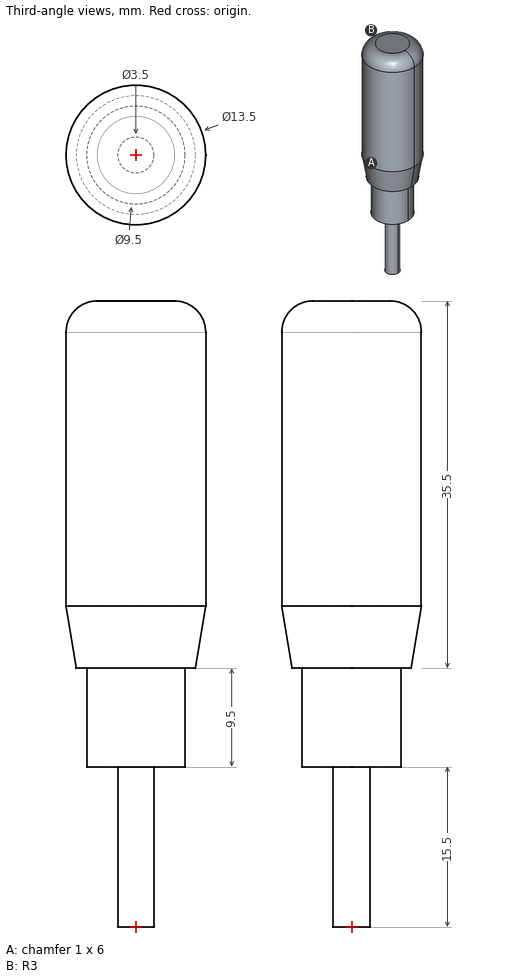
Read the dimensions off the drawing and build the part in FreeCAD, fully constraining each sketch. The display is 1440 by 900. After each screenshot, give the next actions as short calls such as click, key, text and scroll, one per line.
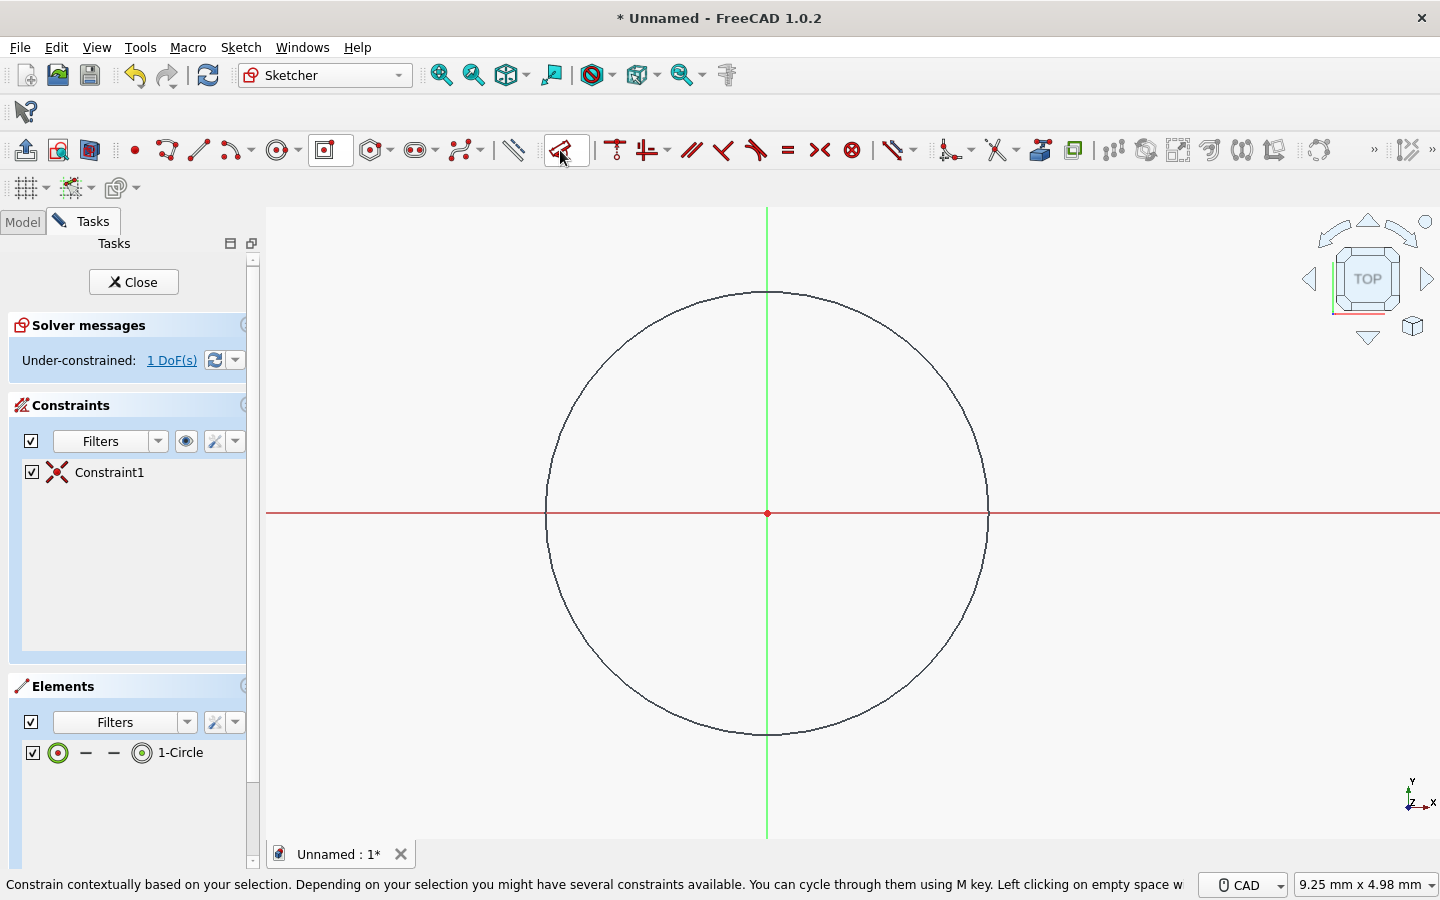
click(923, 356)
click(946, 333)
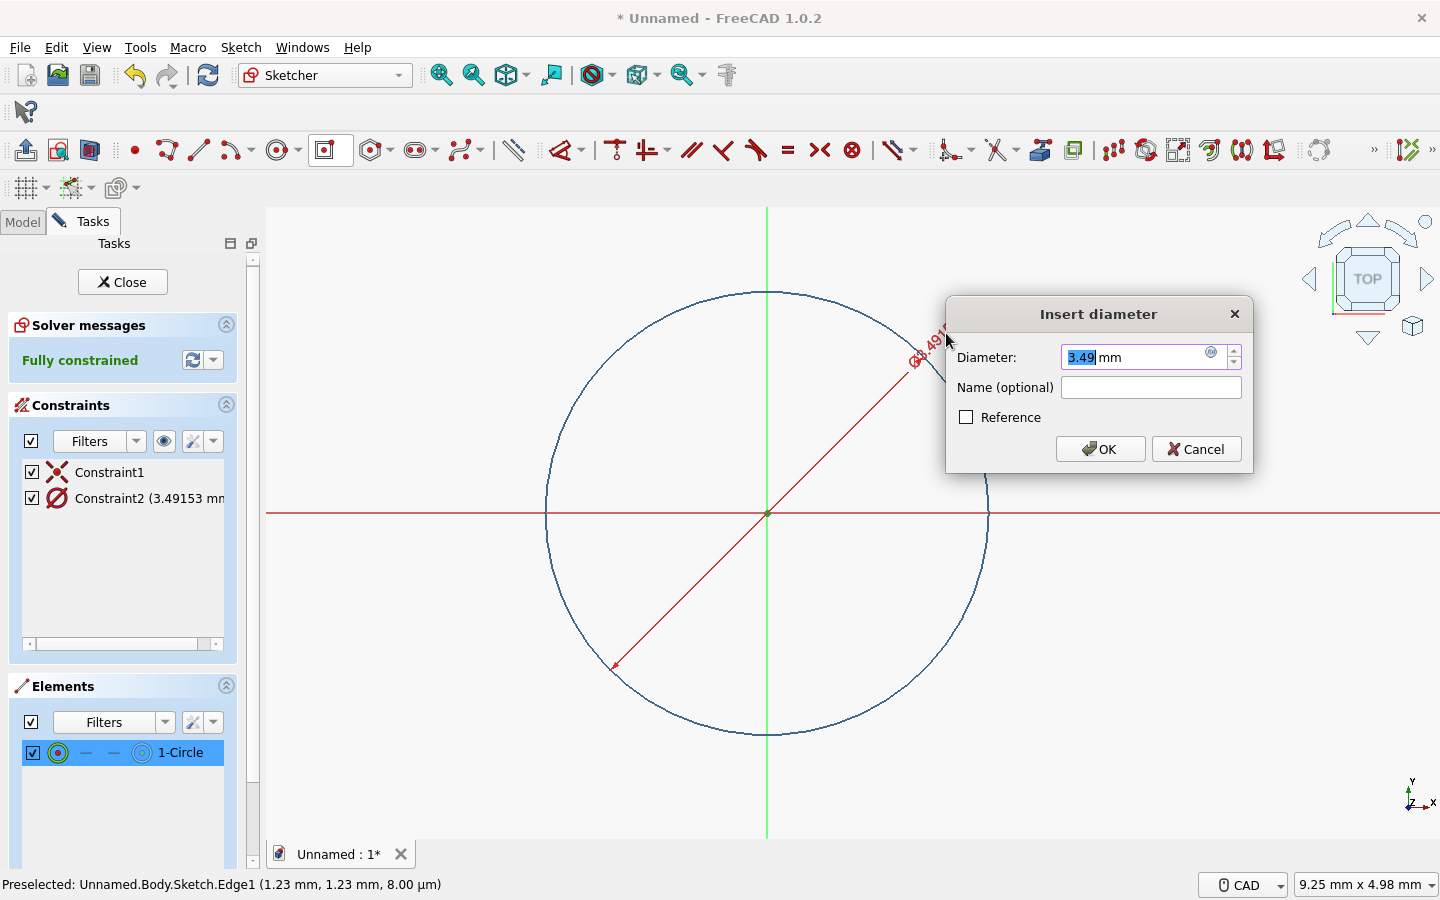
text(3.5)
key(Return)
key(Escape)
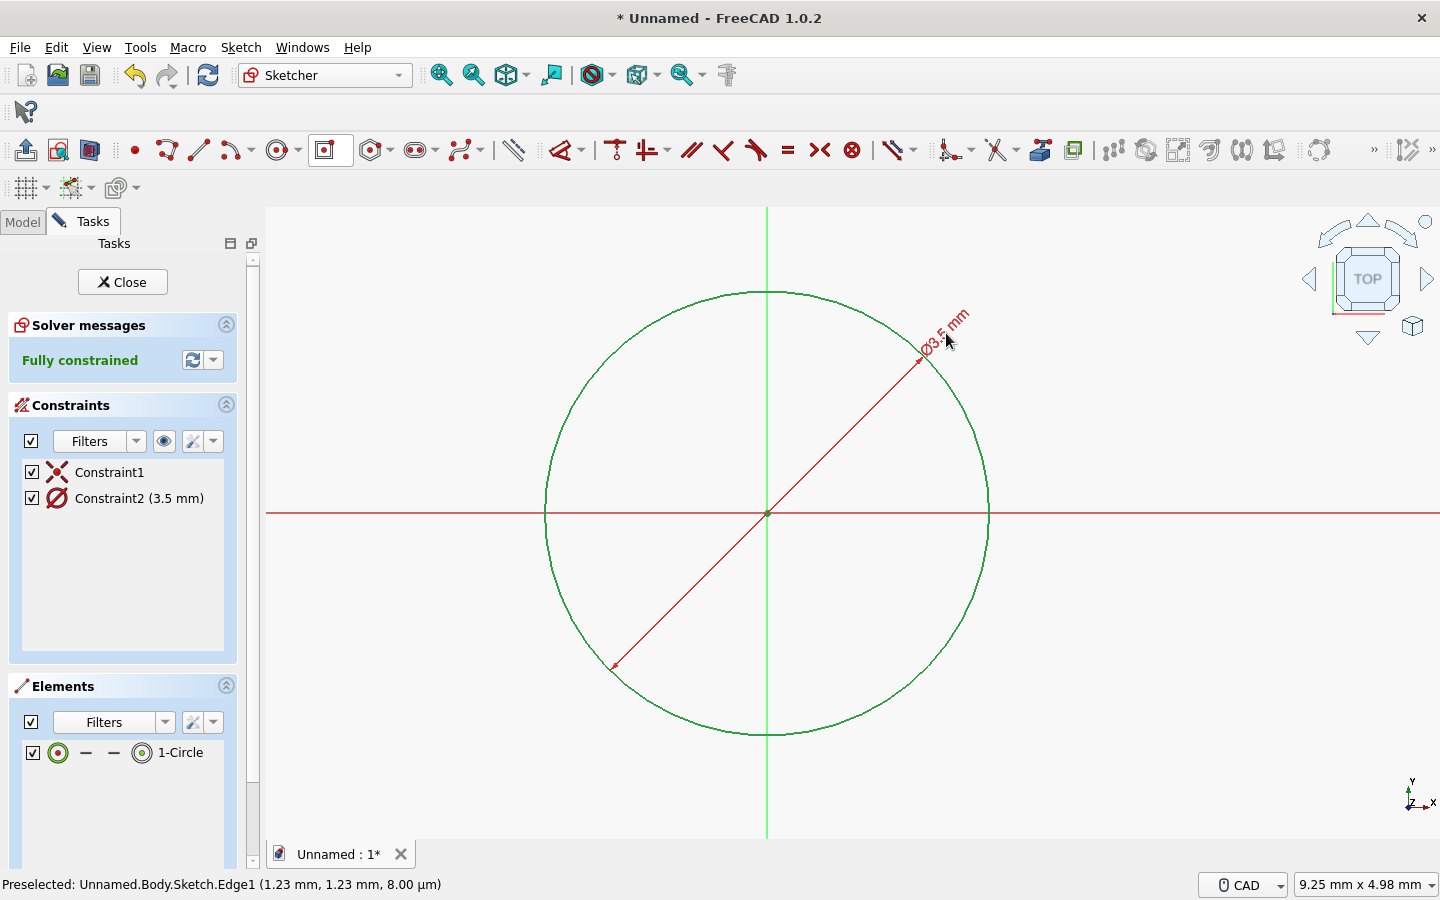
click(123, 282)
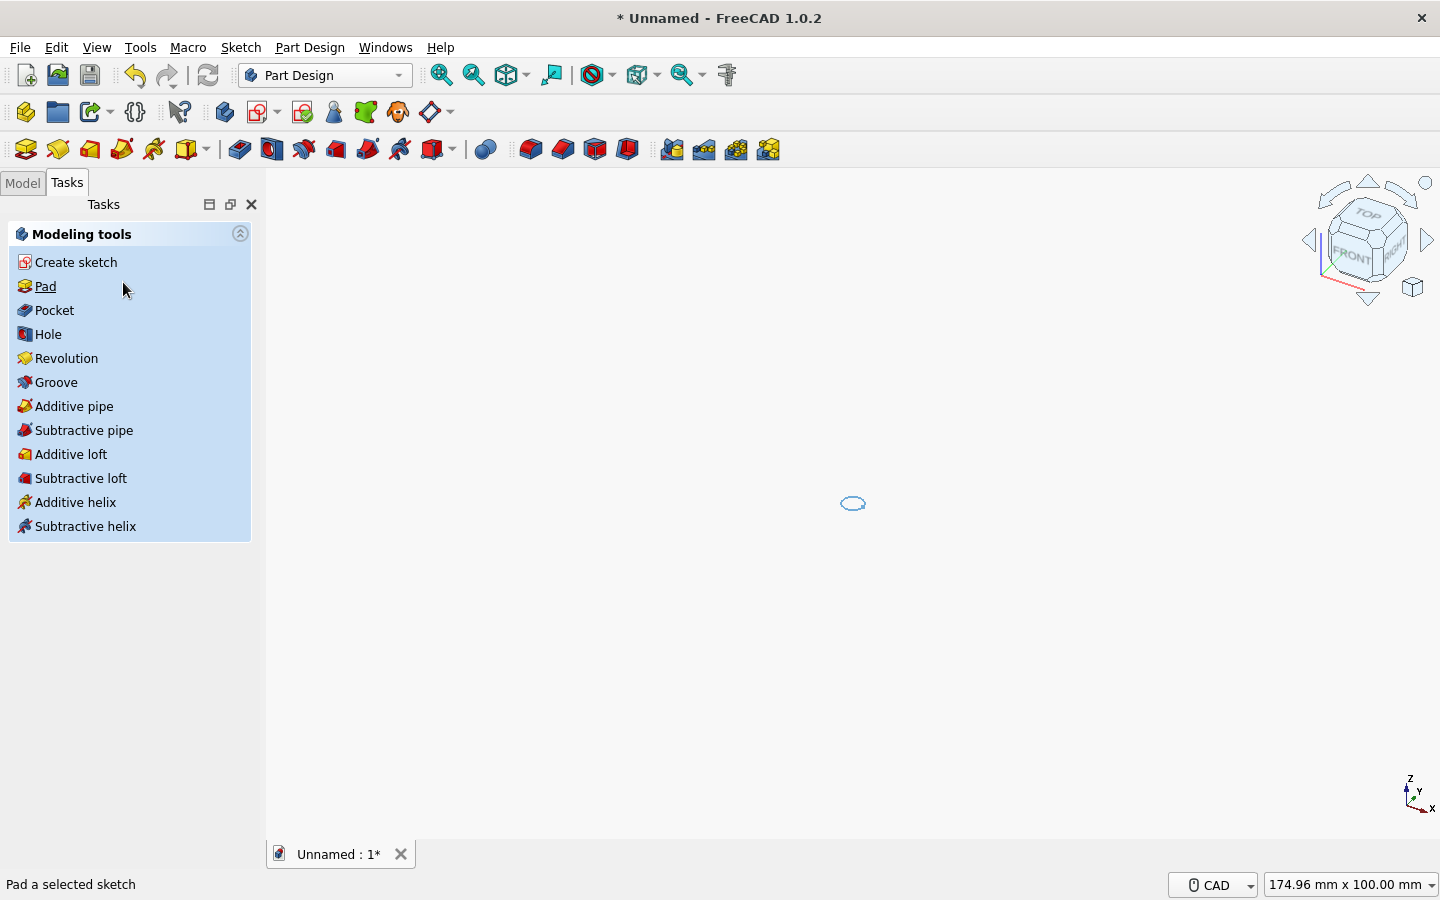
click(26, 150)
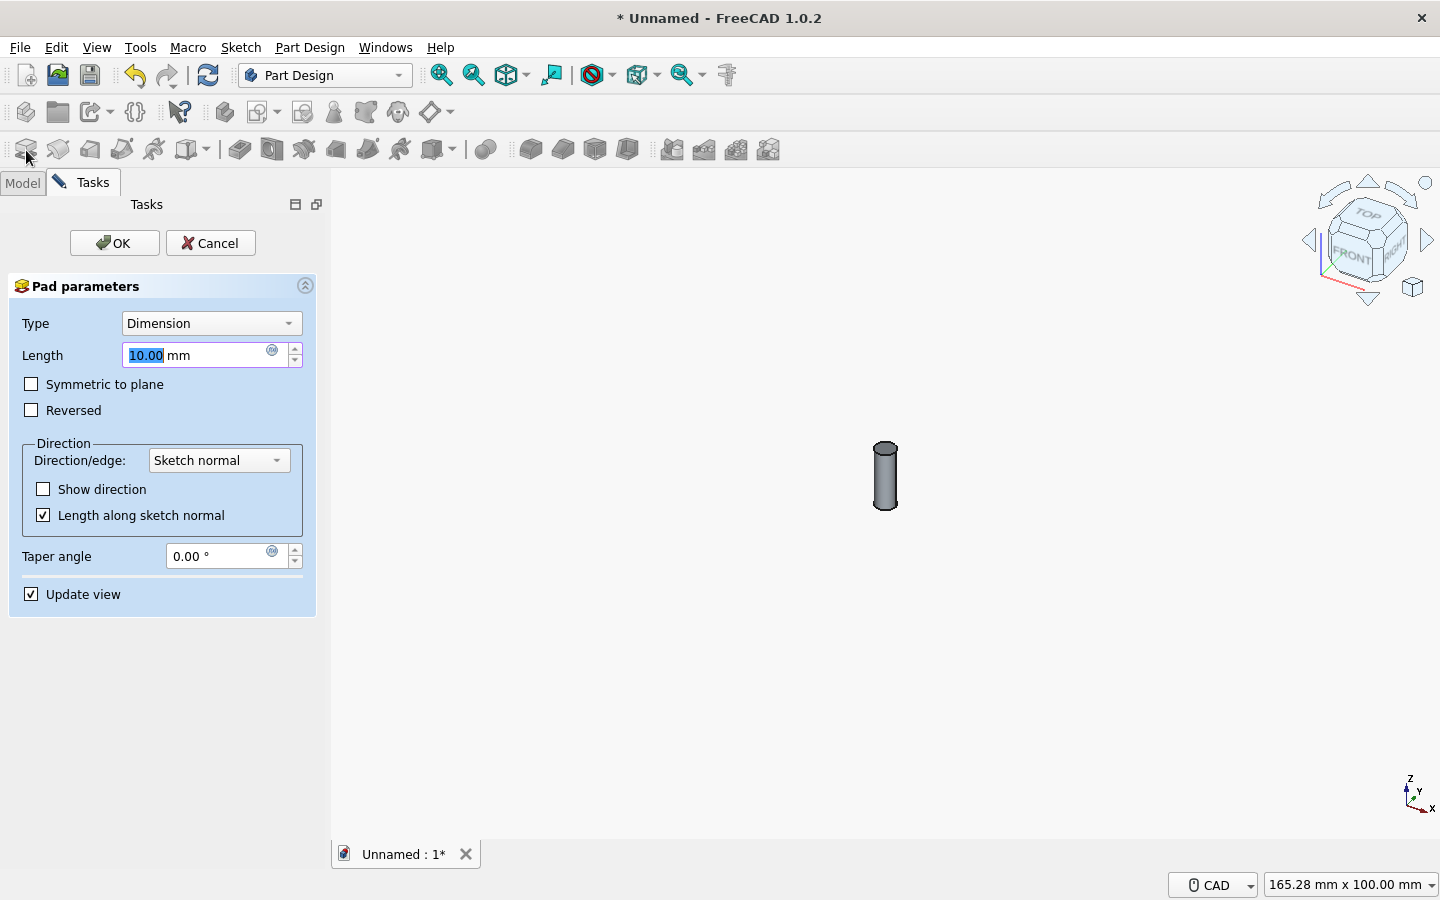
text(15.5)
key(Tab)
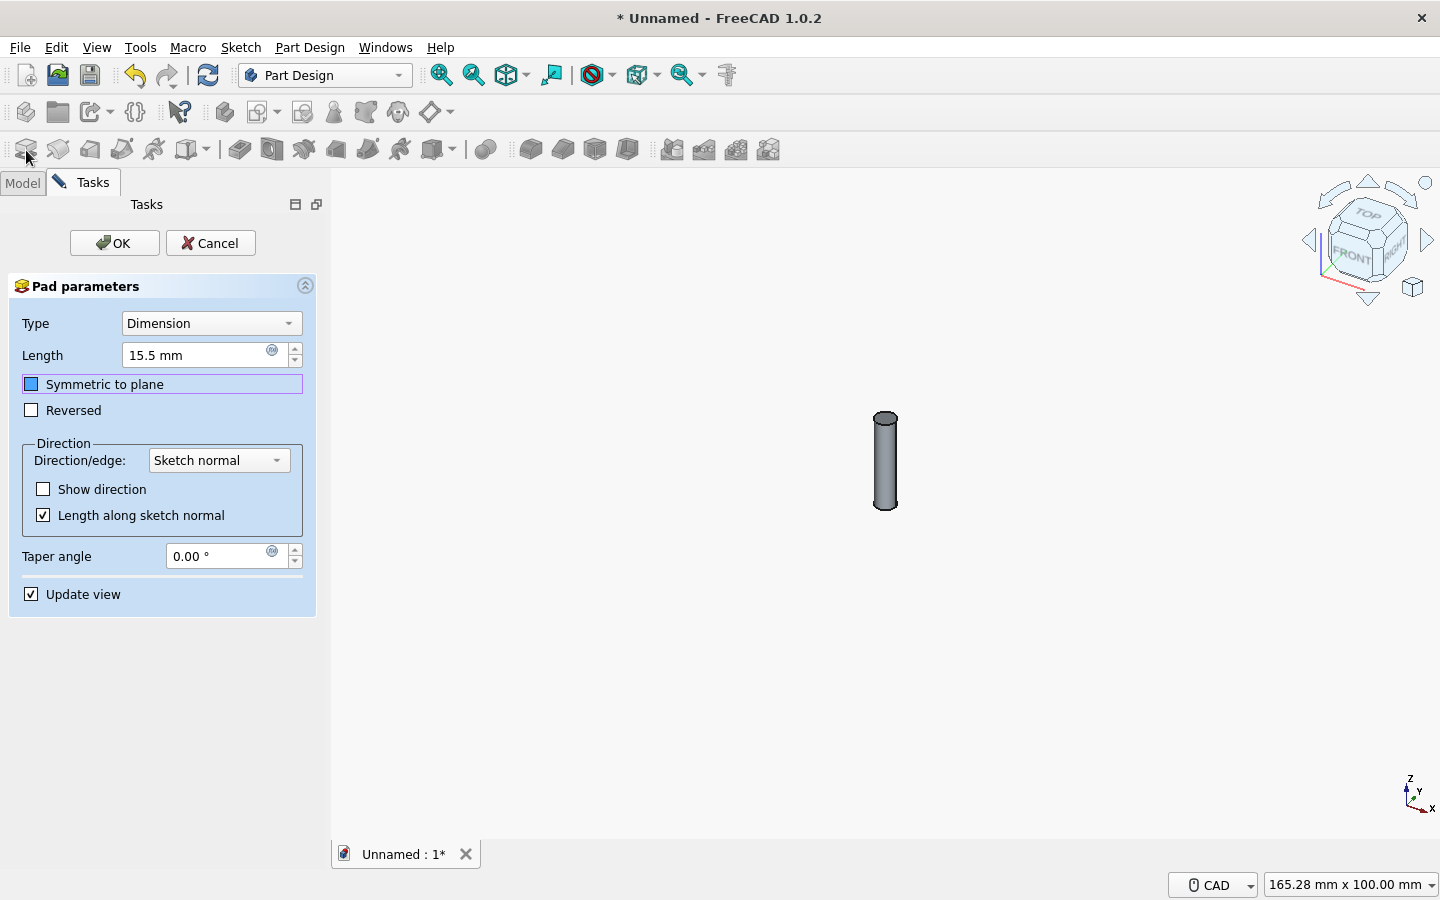
click(115, 243)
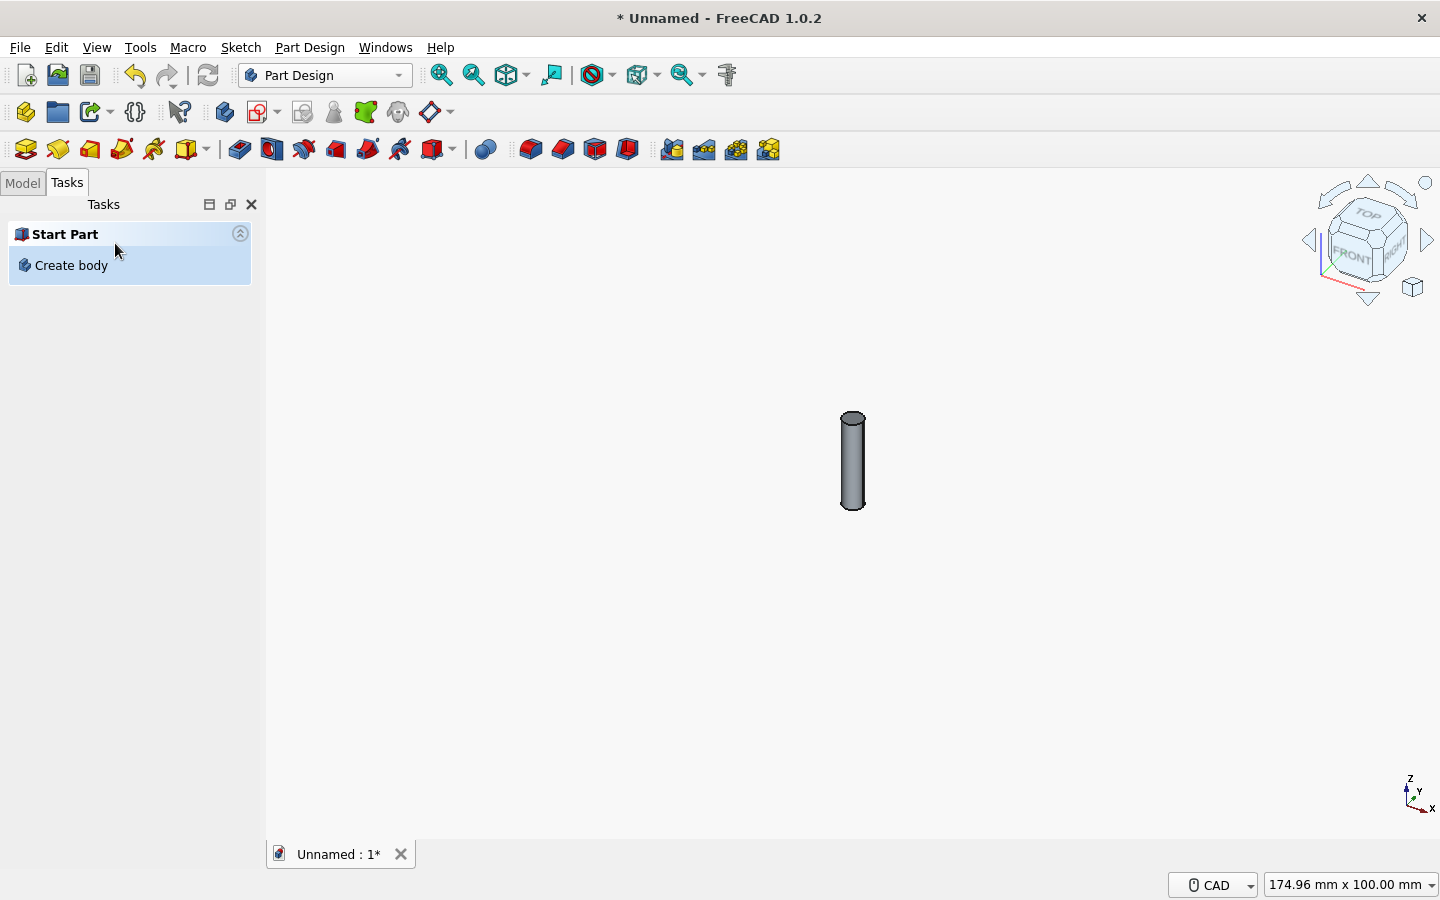
click(442, 76)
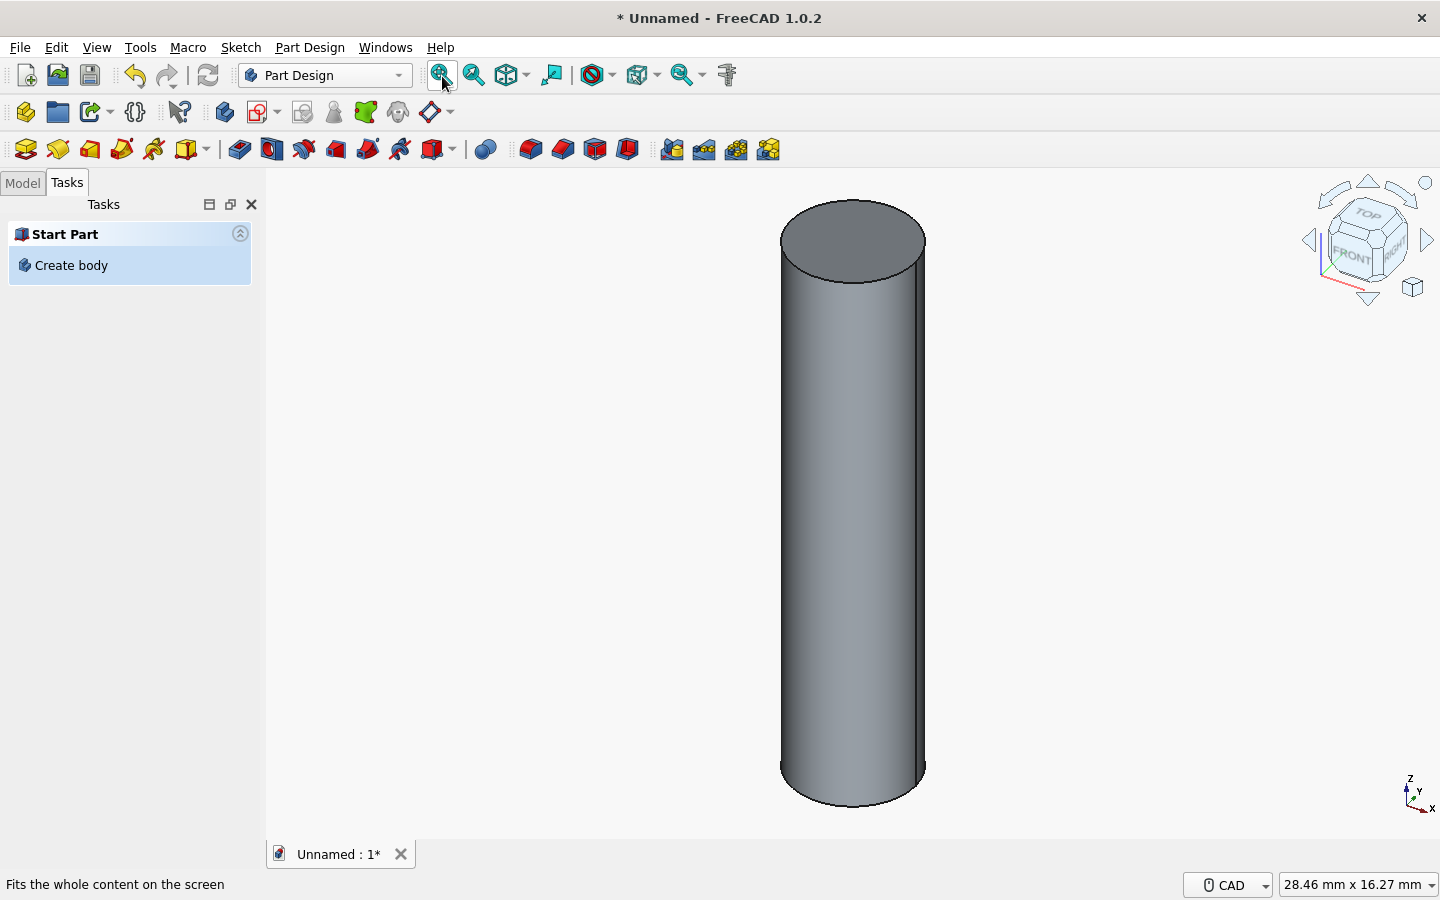
click(853, 241)